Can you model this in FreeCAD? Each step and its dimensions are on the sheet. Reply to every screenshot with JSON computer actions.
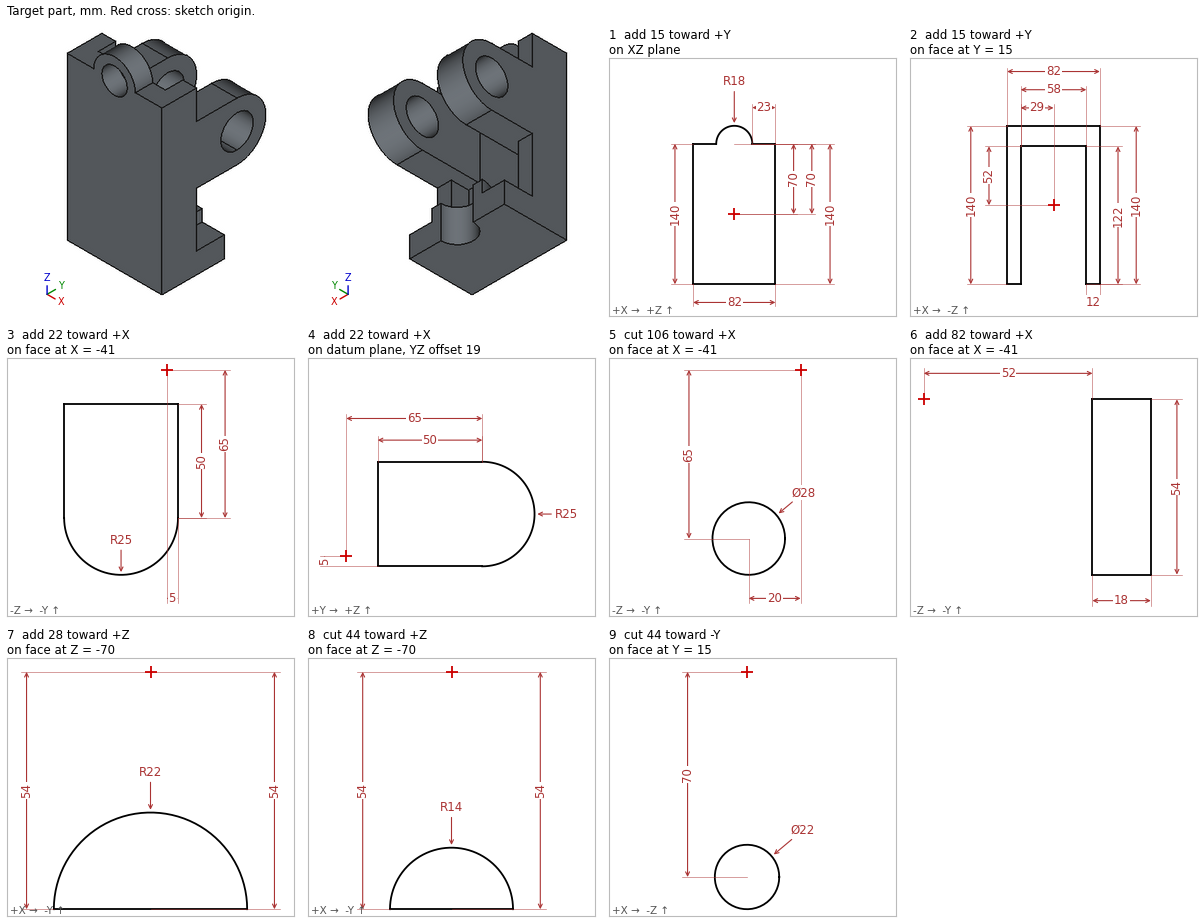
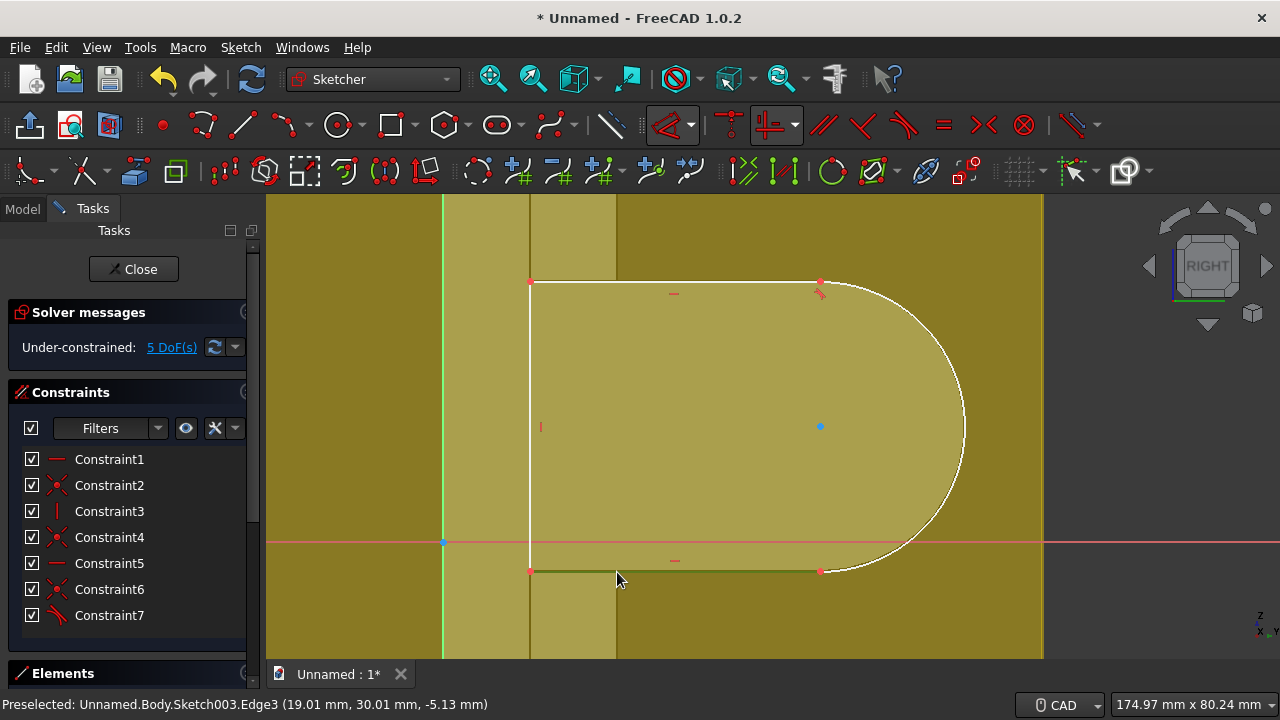
{"action": "left_click", "coordinate": [937, 512]}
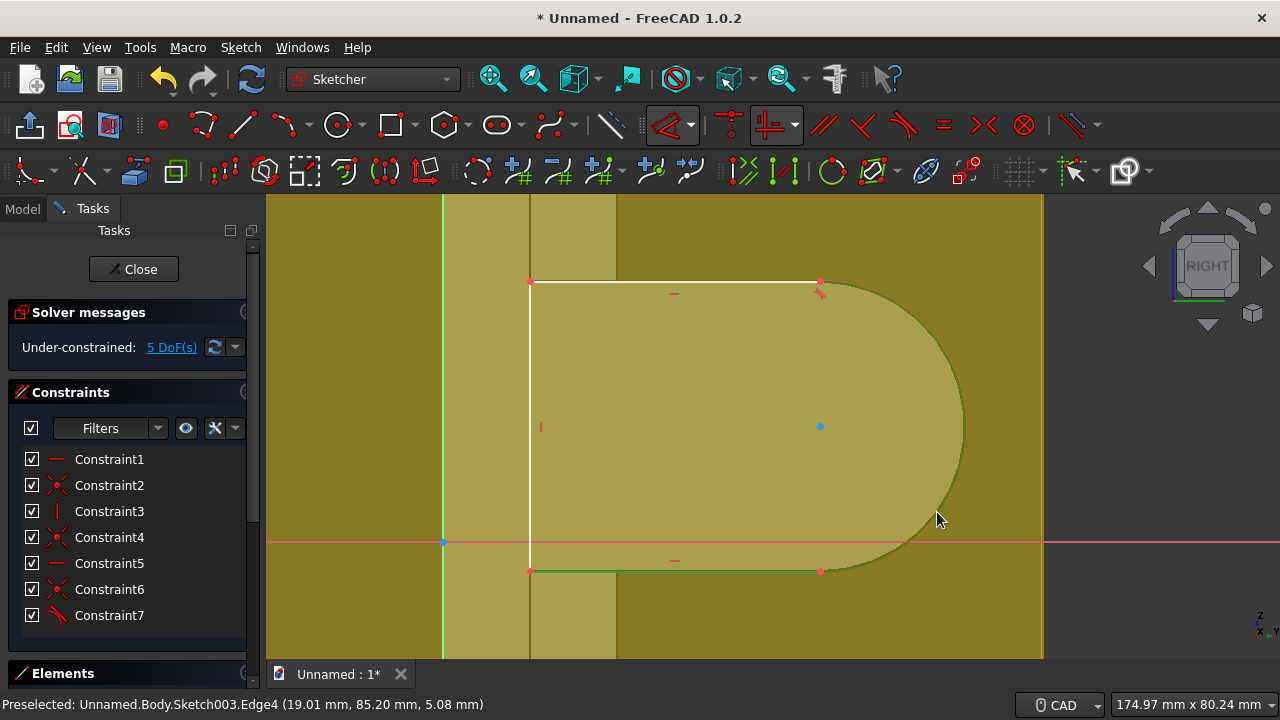
{"action": "left_click", "coordinate": [904, 126]}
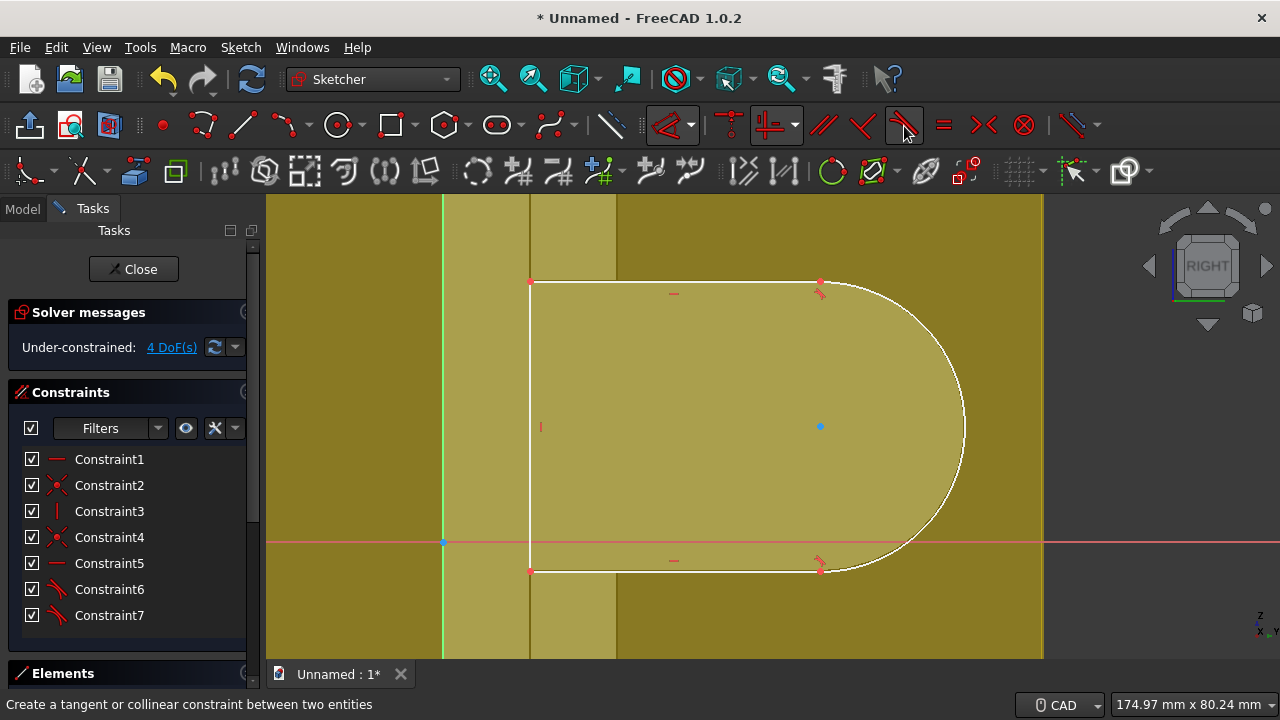
{"action": "left_click", "coordinate": [937, 512]}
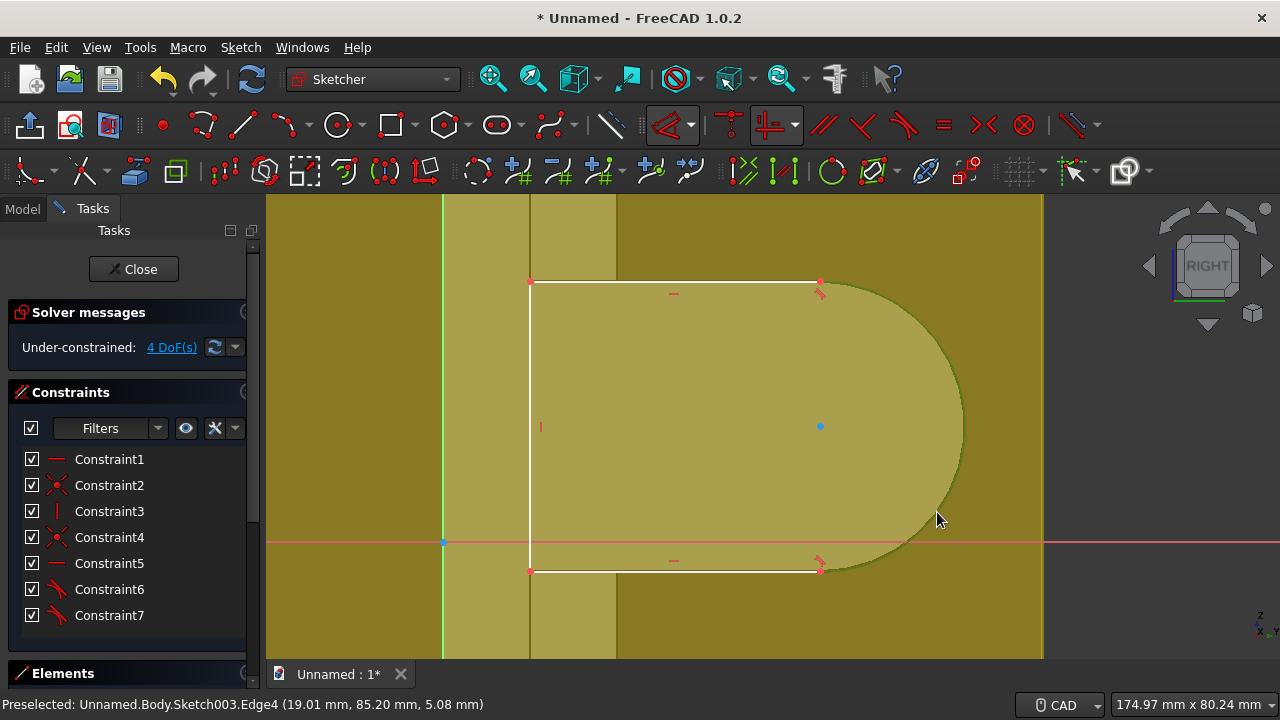
{"action": "key", "text": "k r"}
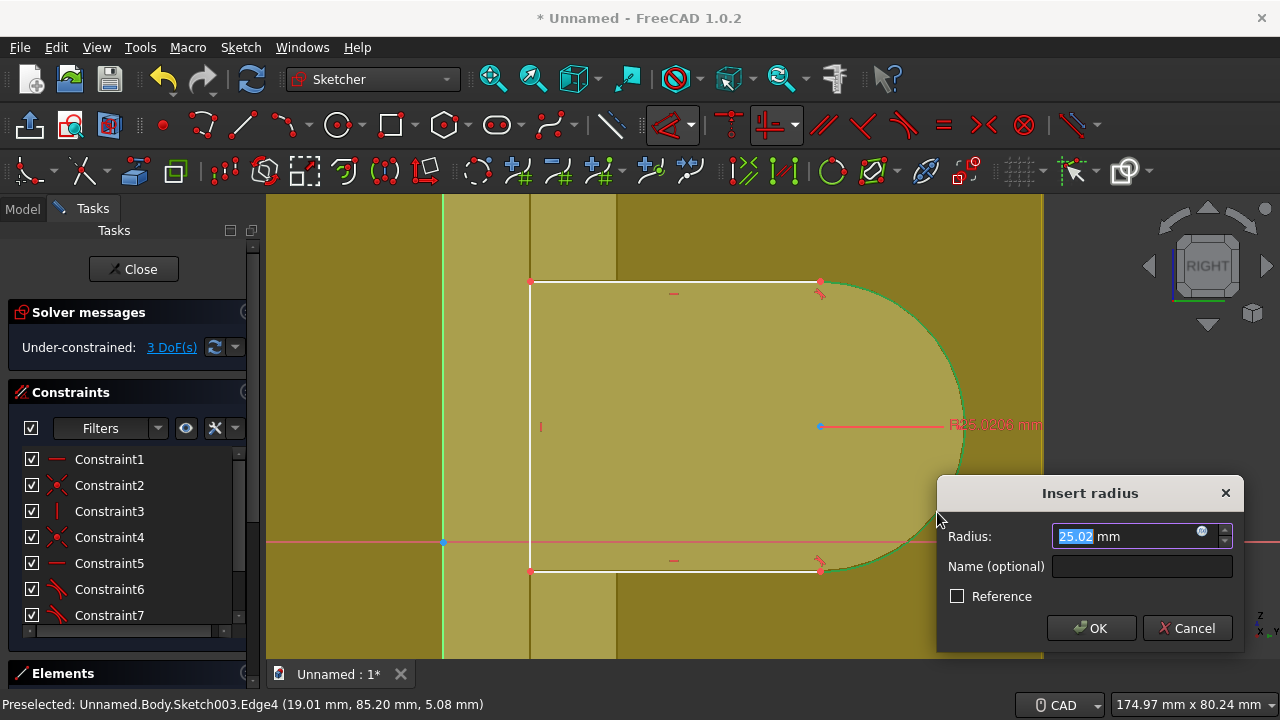
{"action": "type", "text": "25"}
{"action": "key", "text": "Return"}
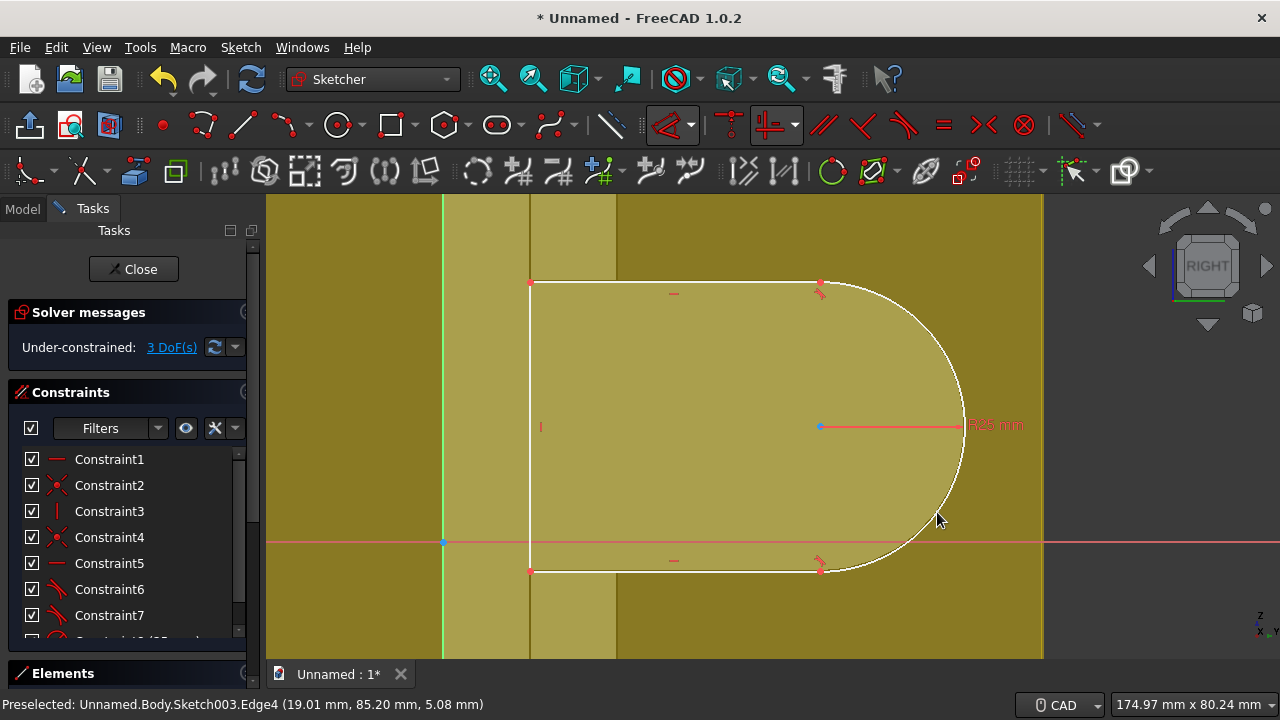
{"action": "left_click", "coordinate": [733, 282]}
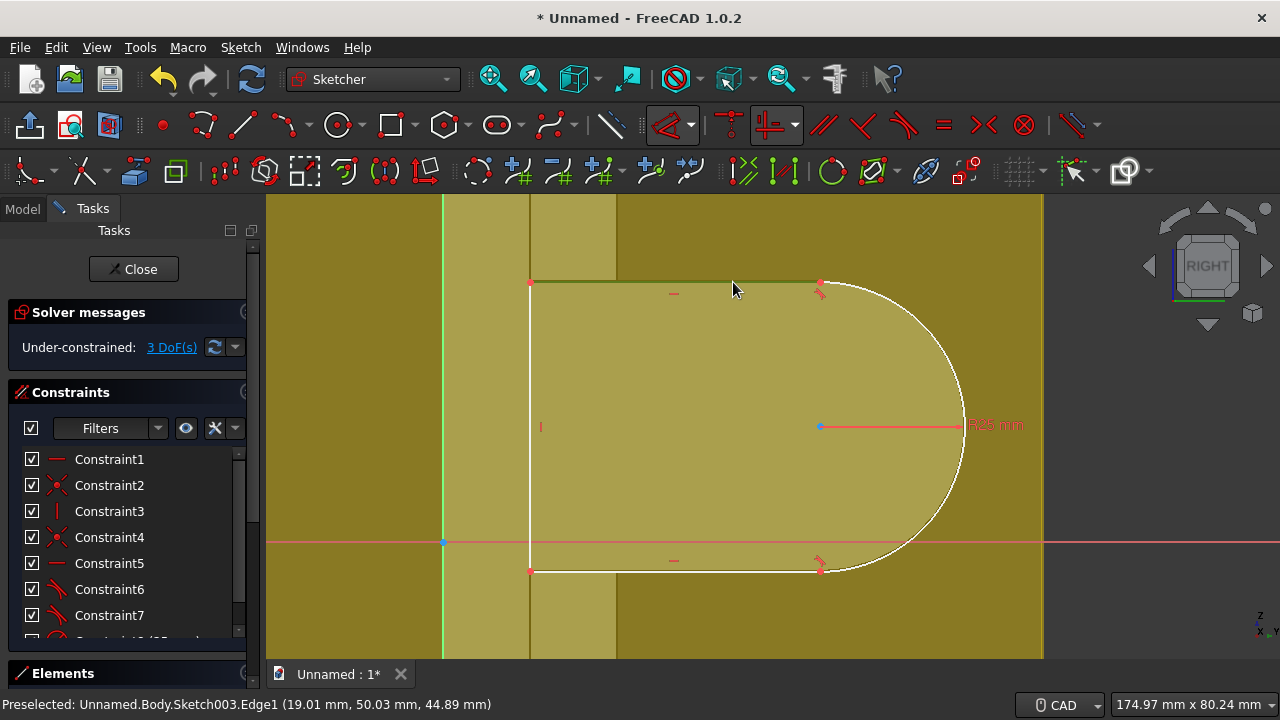
{"action": "key", "text": "l"}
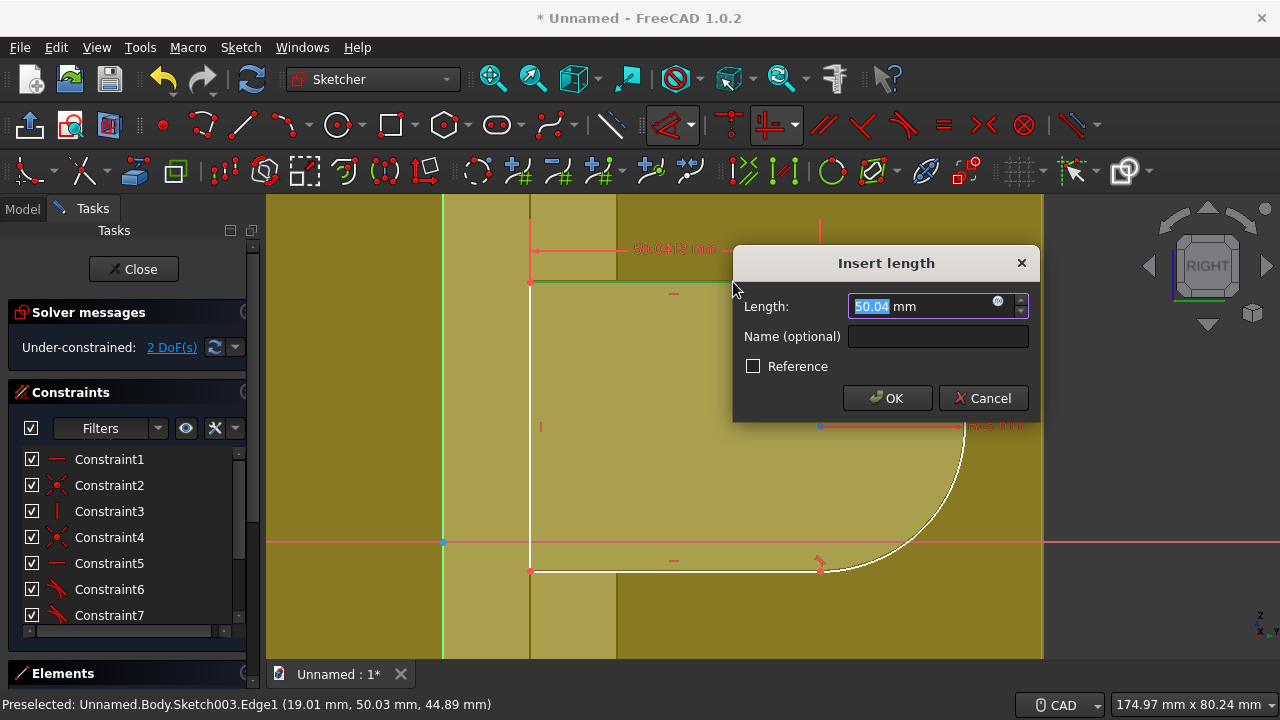
{"action": "type", "text": "50"}
{"action": "key", "text": "Return"}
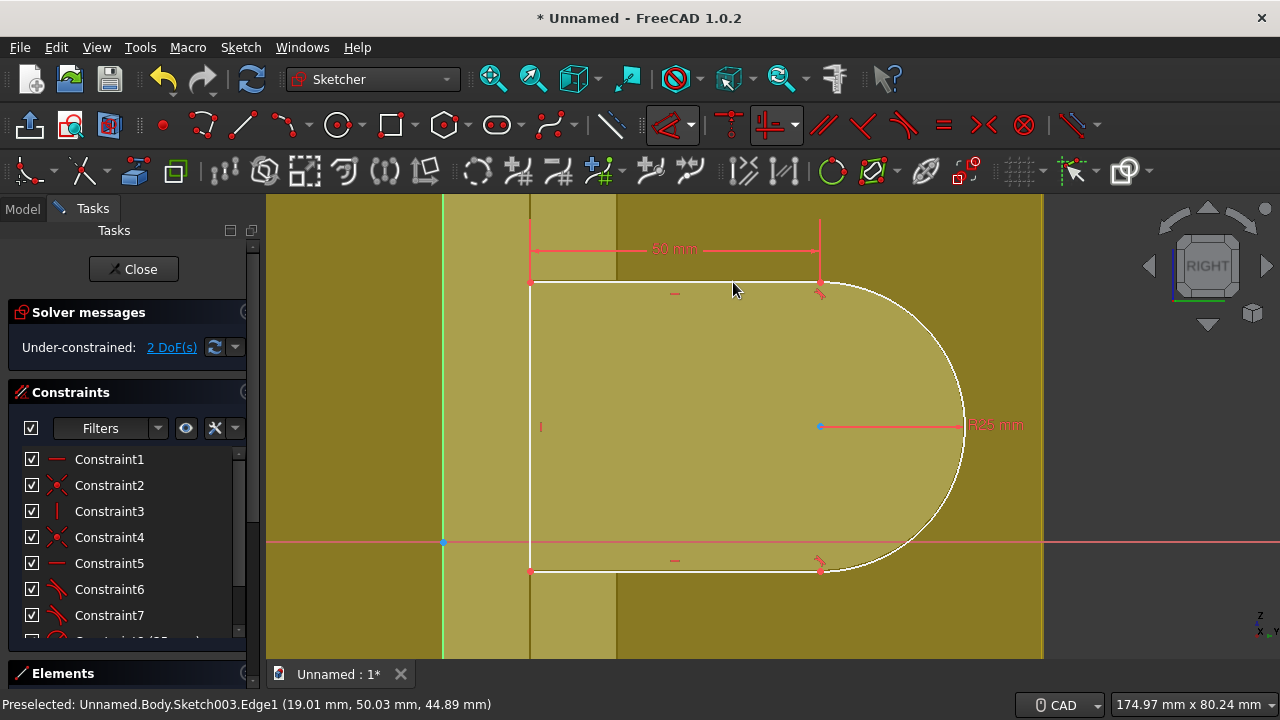
{"action": "scroll", "coordinate": [530, 572], "scroll_direction": "up", "scroll_amount": 2}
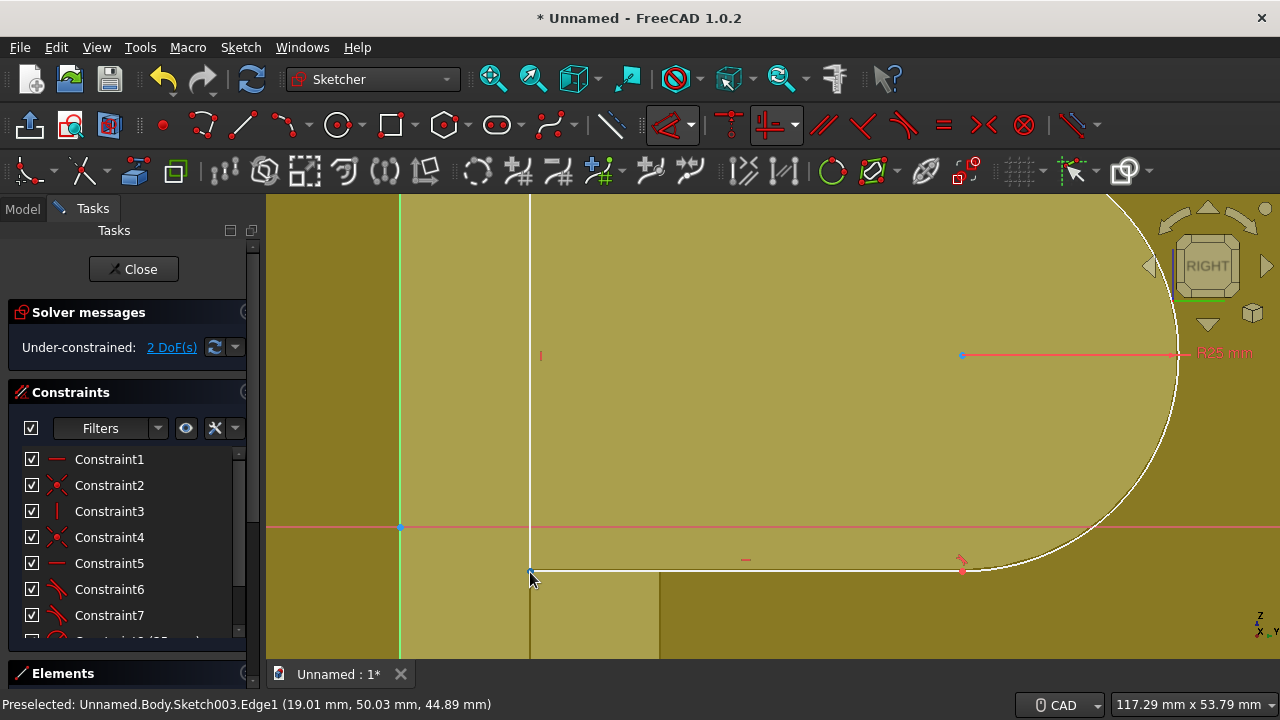
{"action": "left_click", "coordinate": [530, 571]}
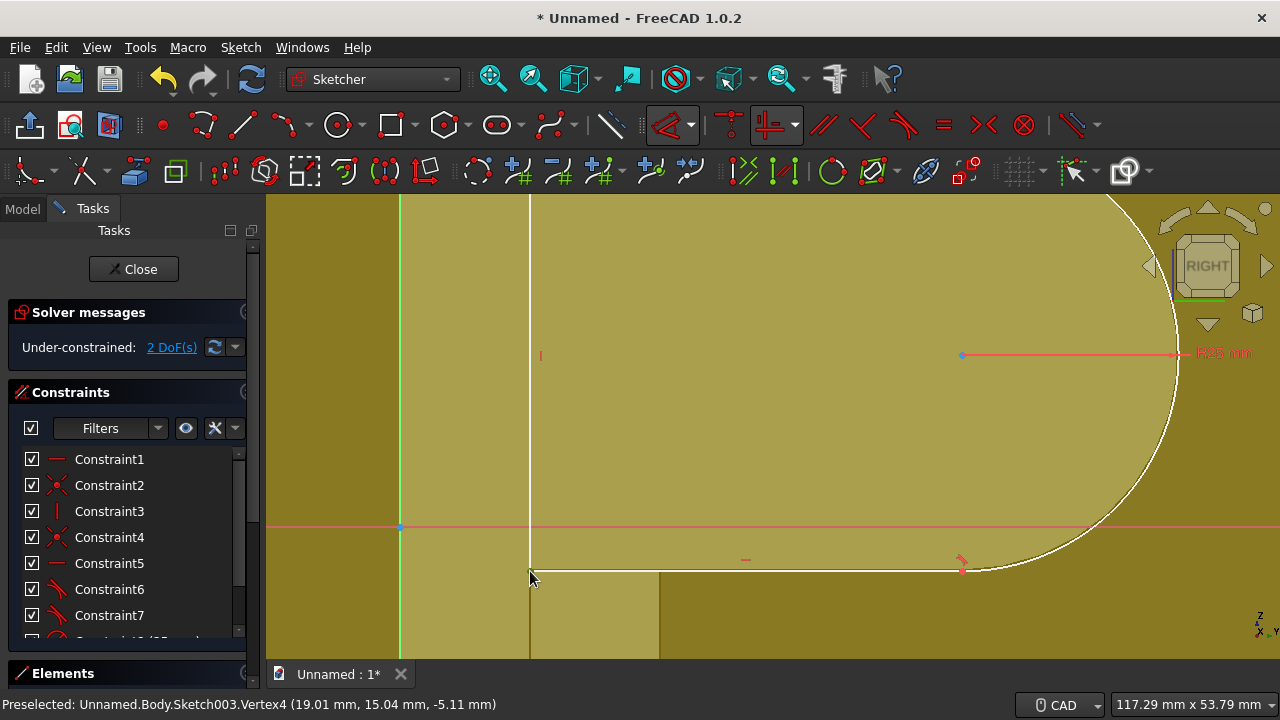
{"action": "key", "text": "i"}